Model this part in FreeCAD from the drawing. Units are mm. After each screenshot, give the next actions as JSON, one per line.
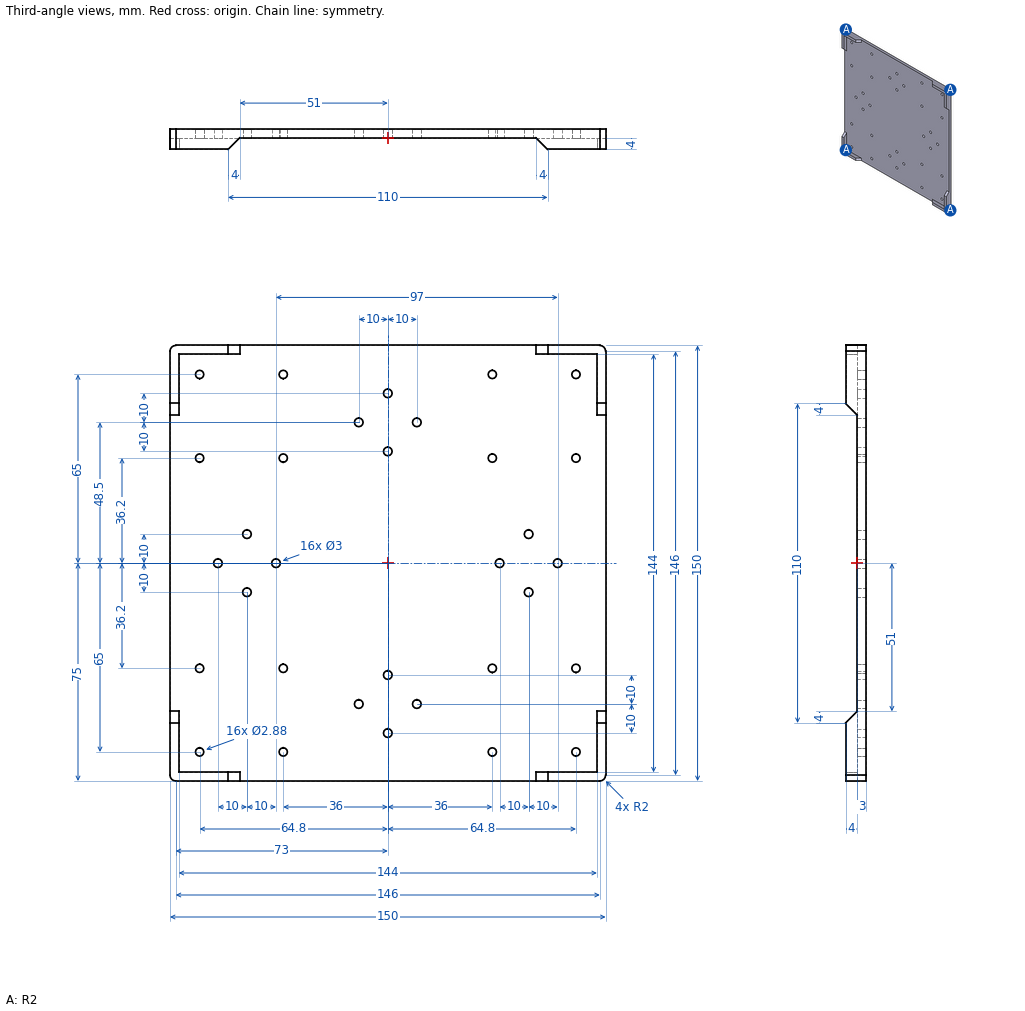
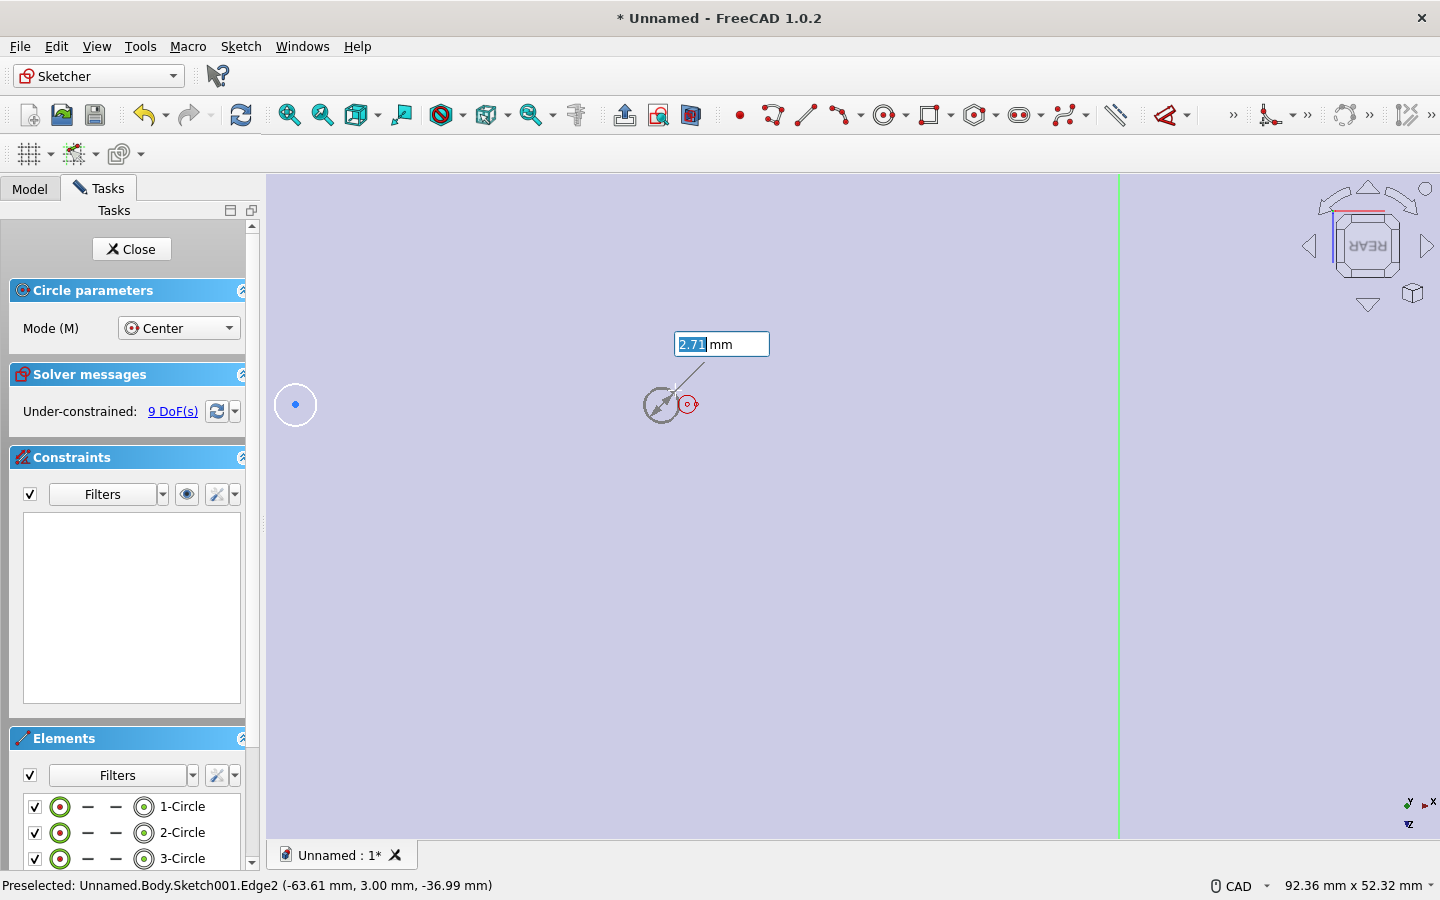
{"action": "left_click", "coordinate": [674, 388]}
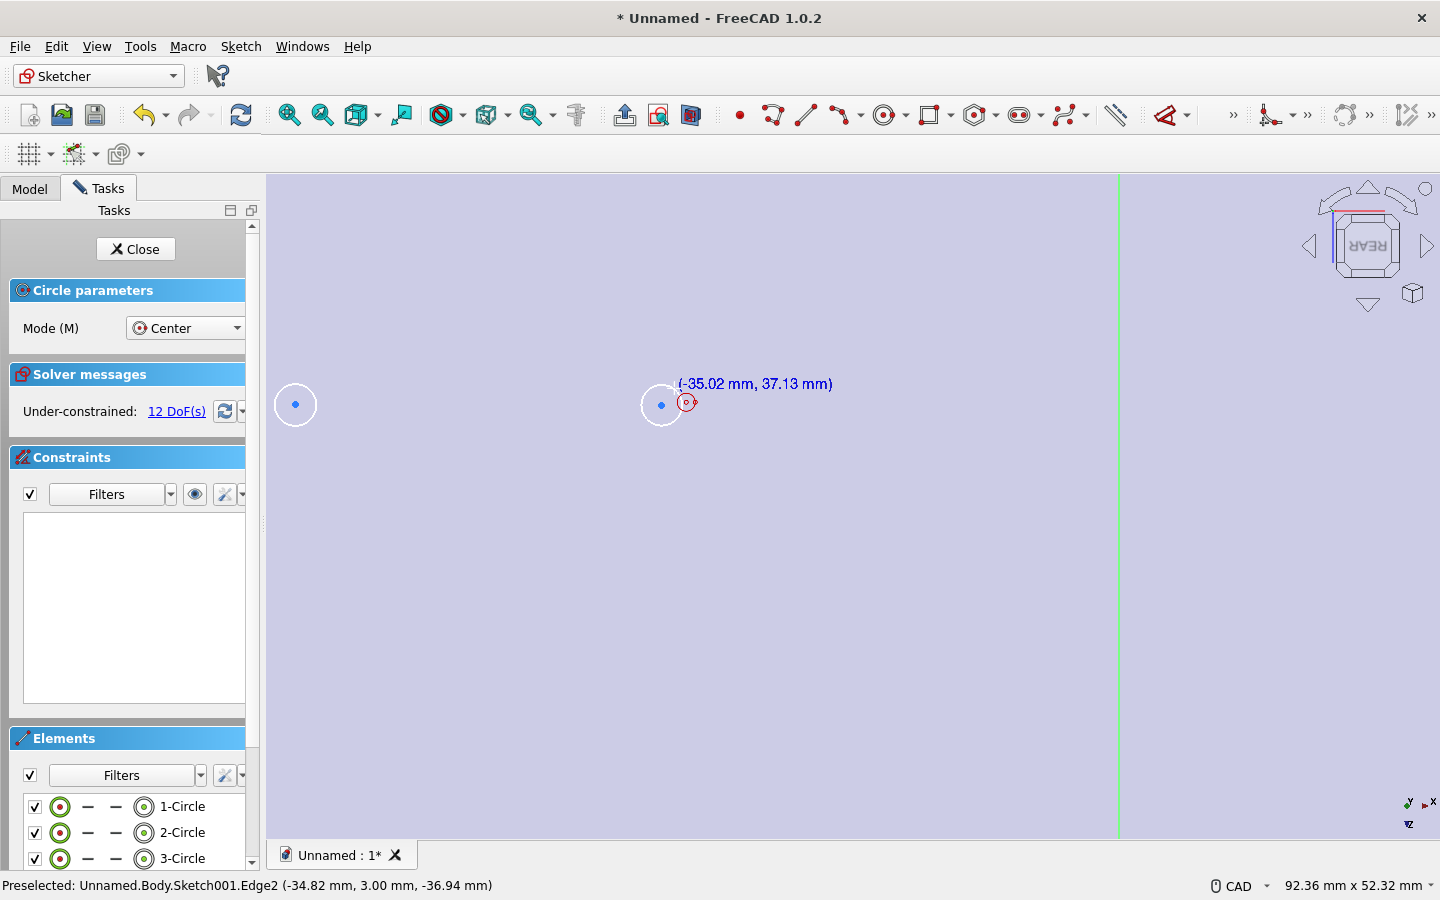
{"action": "scroll", "coordinate": [675, 390], "scroll_direction": "down", "scroll_amount": 7}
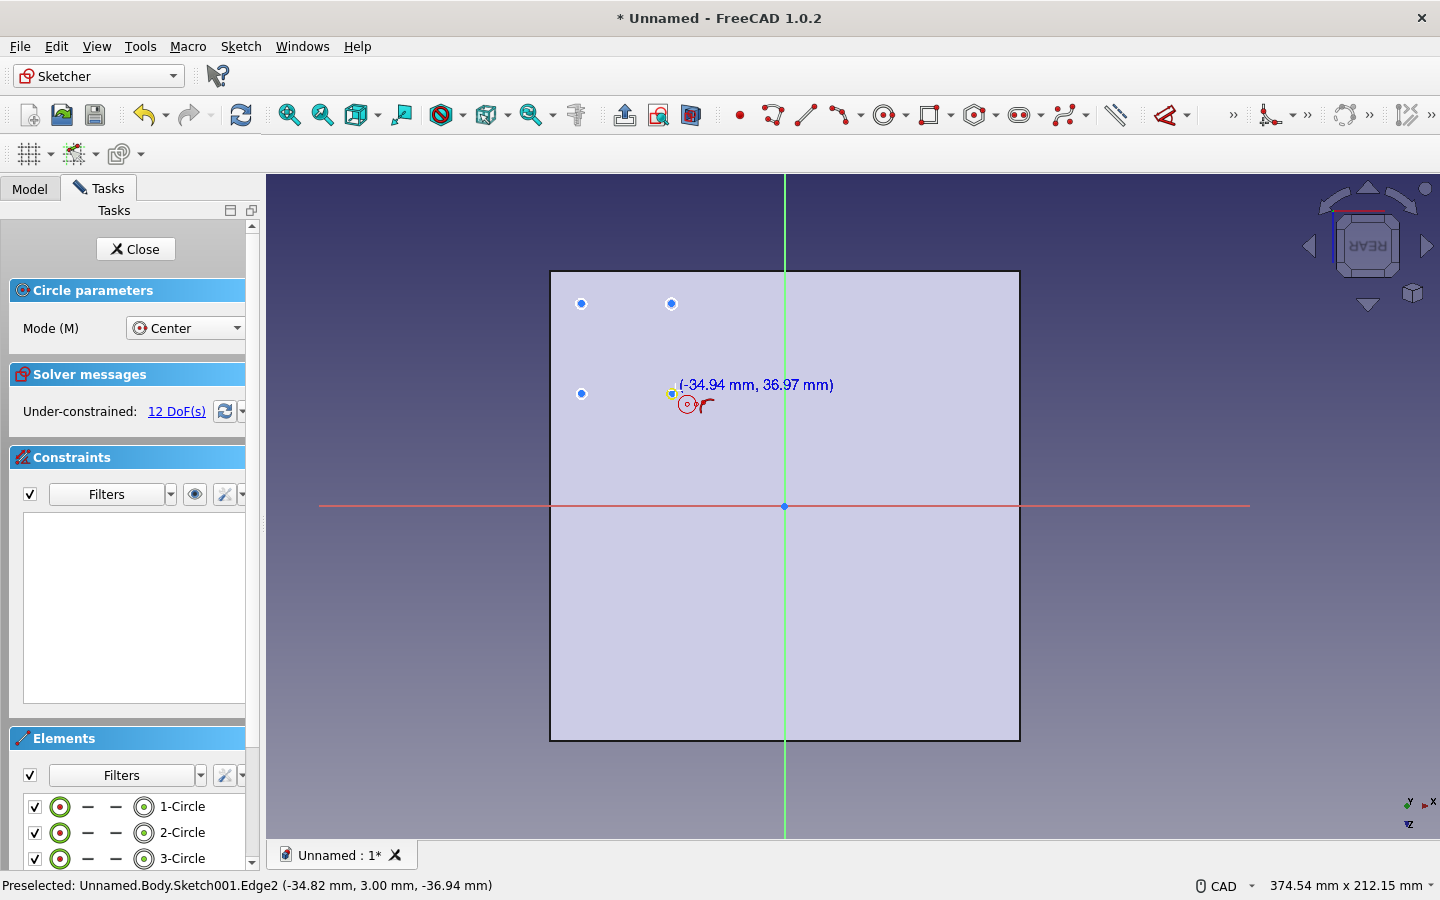
{"action": "scroll", "coordinate": [898, 303], "scroll_direction": "up", "scroll_amount": 9}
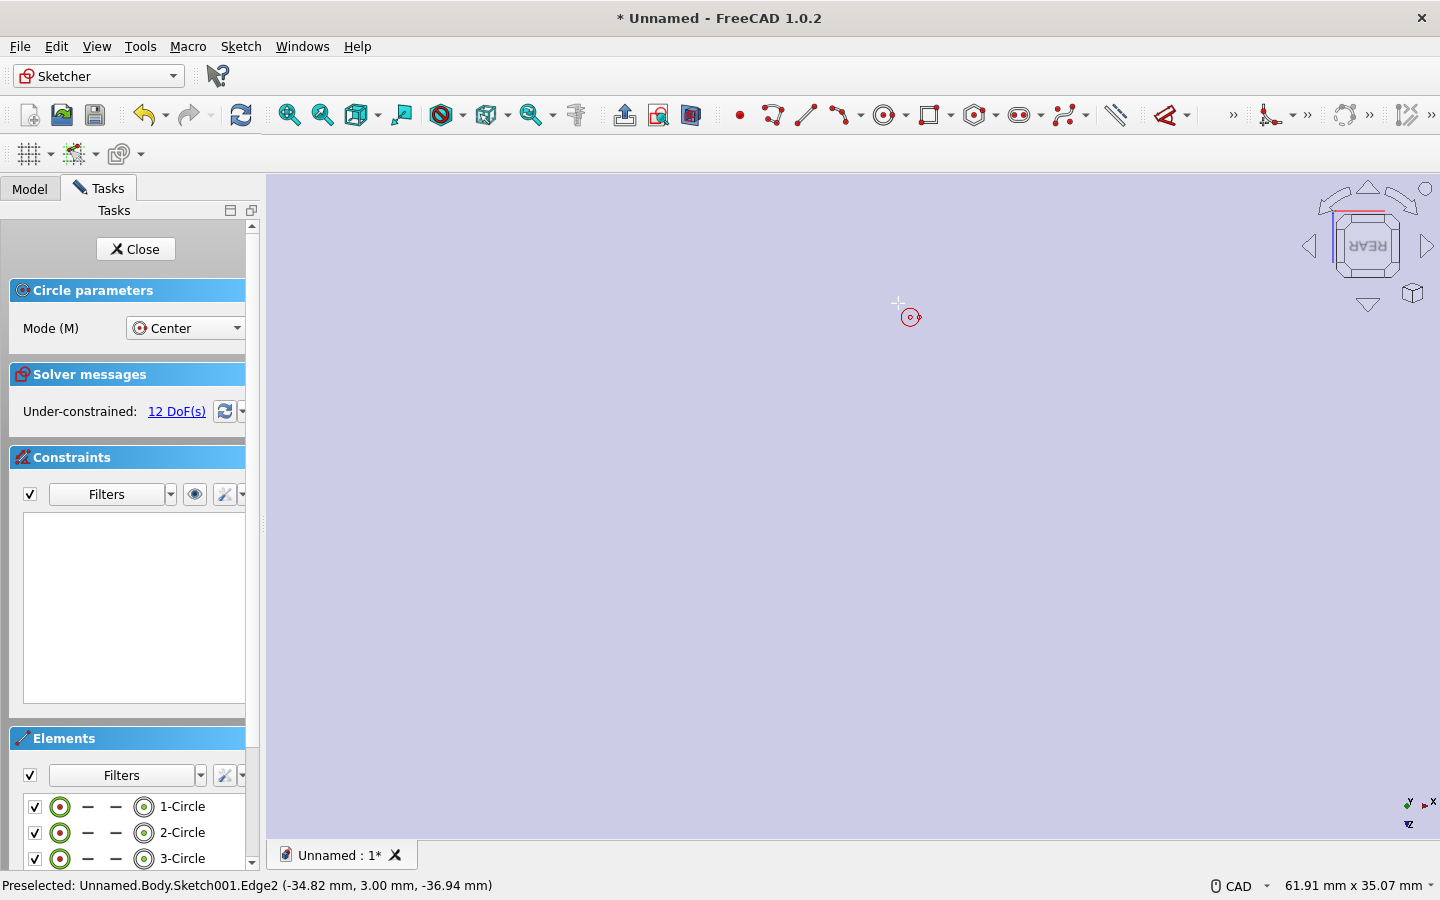
{"action": "scroll", "coordinate": [898, 303], "scroll_direction": "down", "scroll_amount": 9}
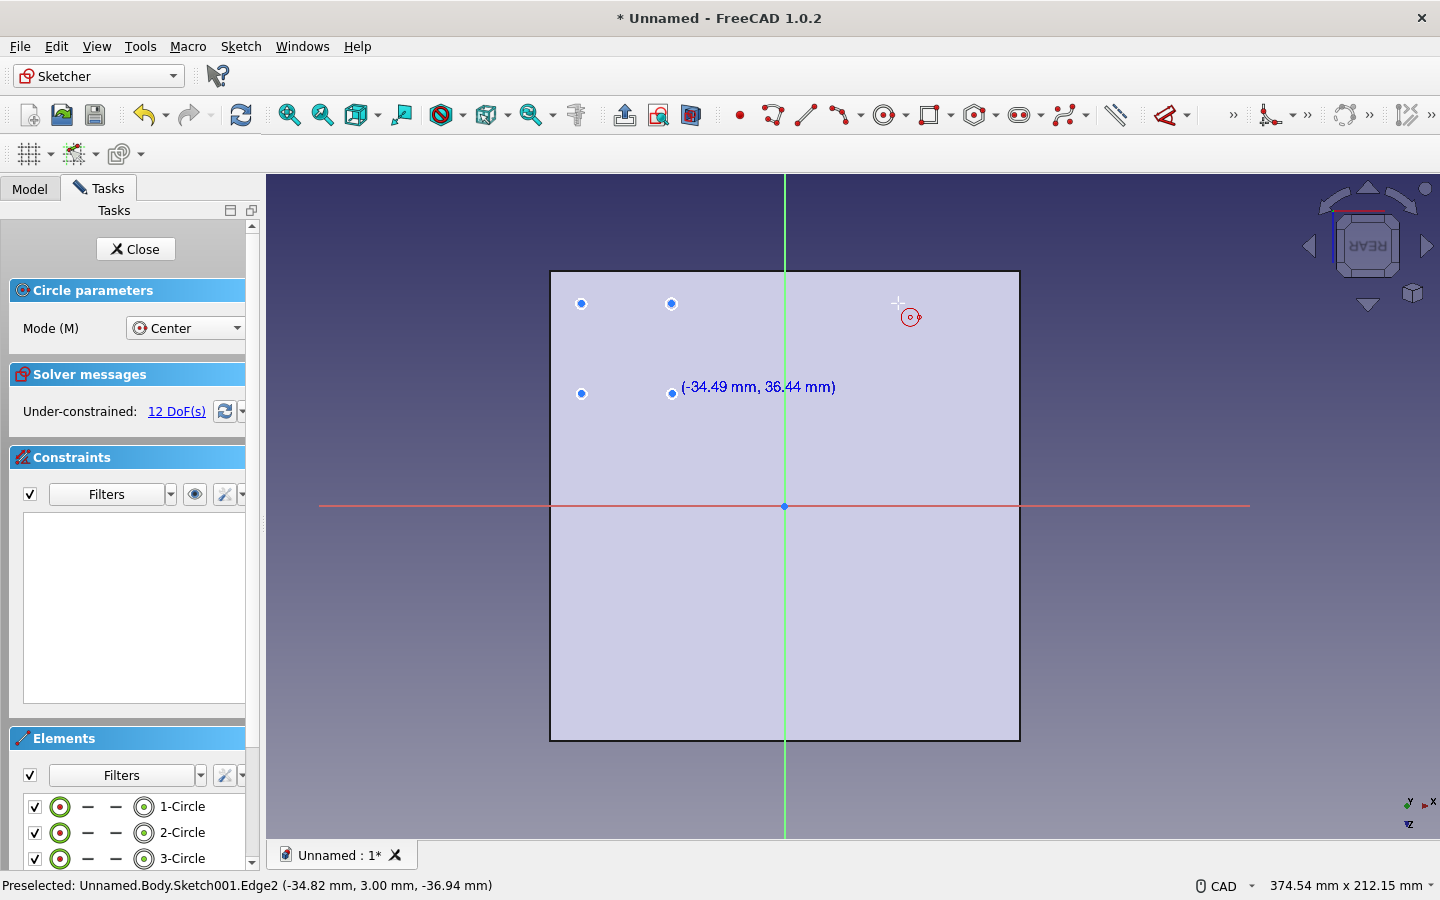
{"action": "left_click", "coordinate": [898, 303]}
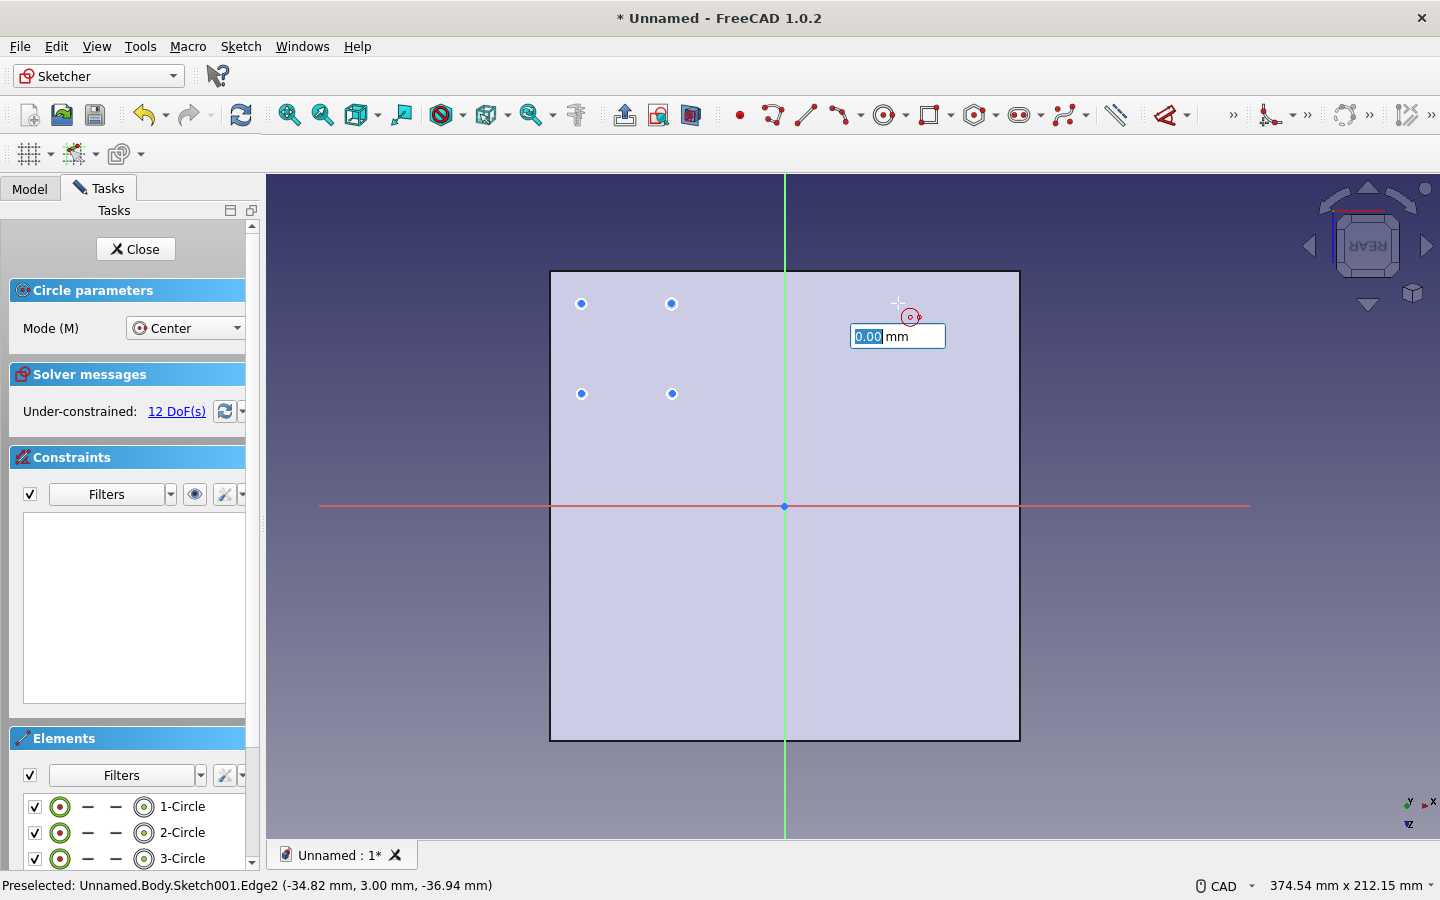
{"action": "scroll", "coordinate": [901, 299], "scroll_direction": "up", "scroll_amount": 7}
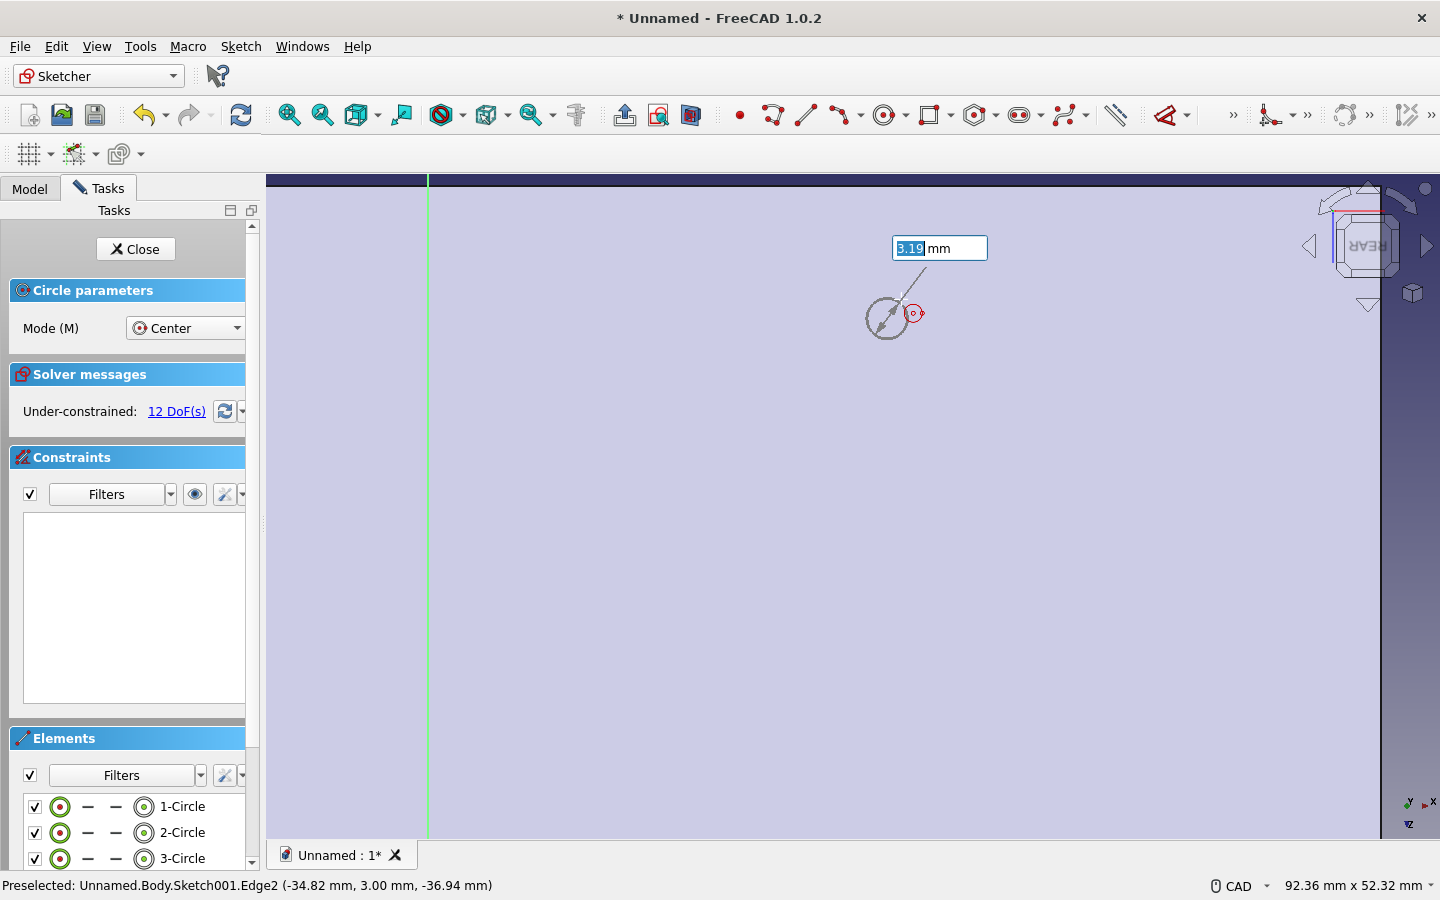
{"action": "left_click", "coordinate": [899, 300]}